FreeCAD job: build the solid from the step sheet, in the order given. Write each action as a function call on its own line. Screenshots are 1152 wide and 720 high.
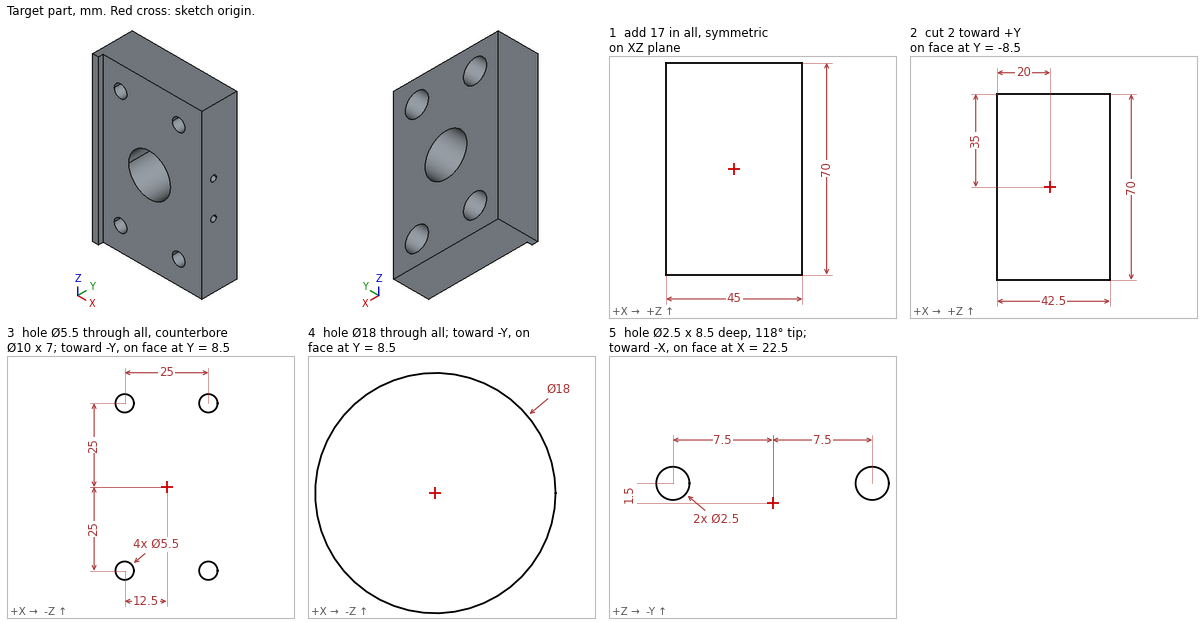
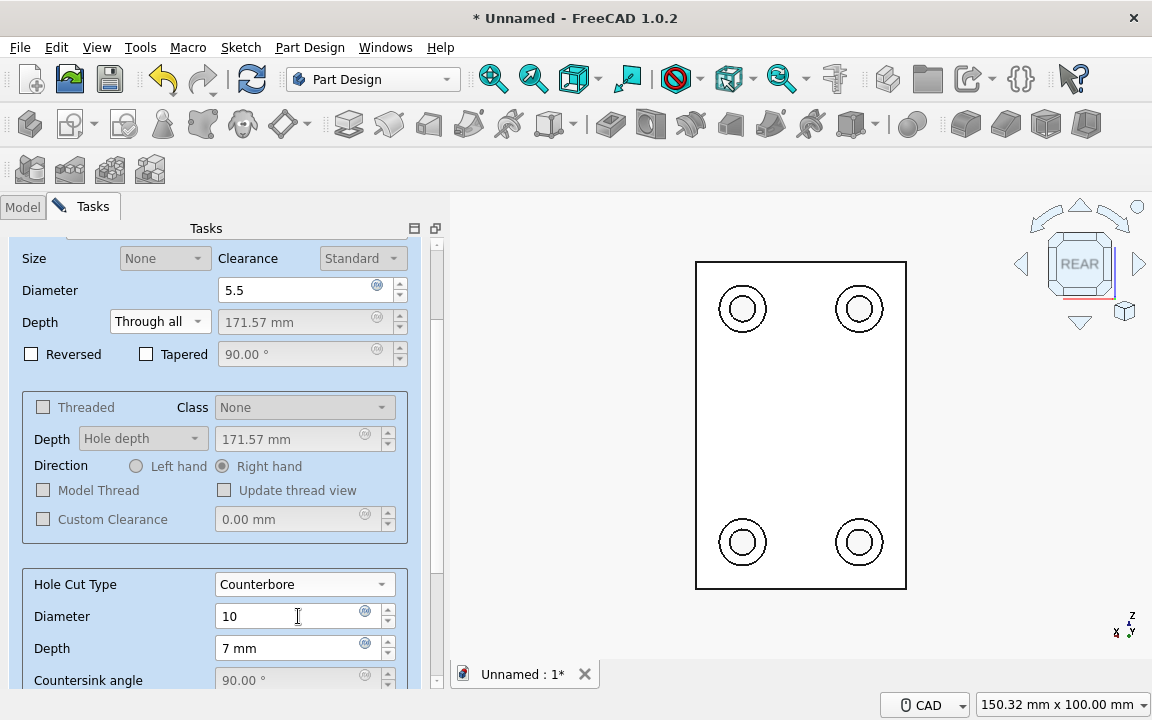
scroll(437, 463, up, 3)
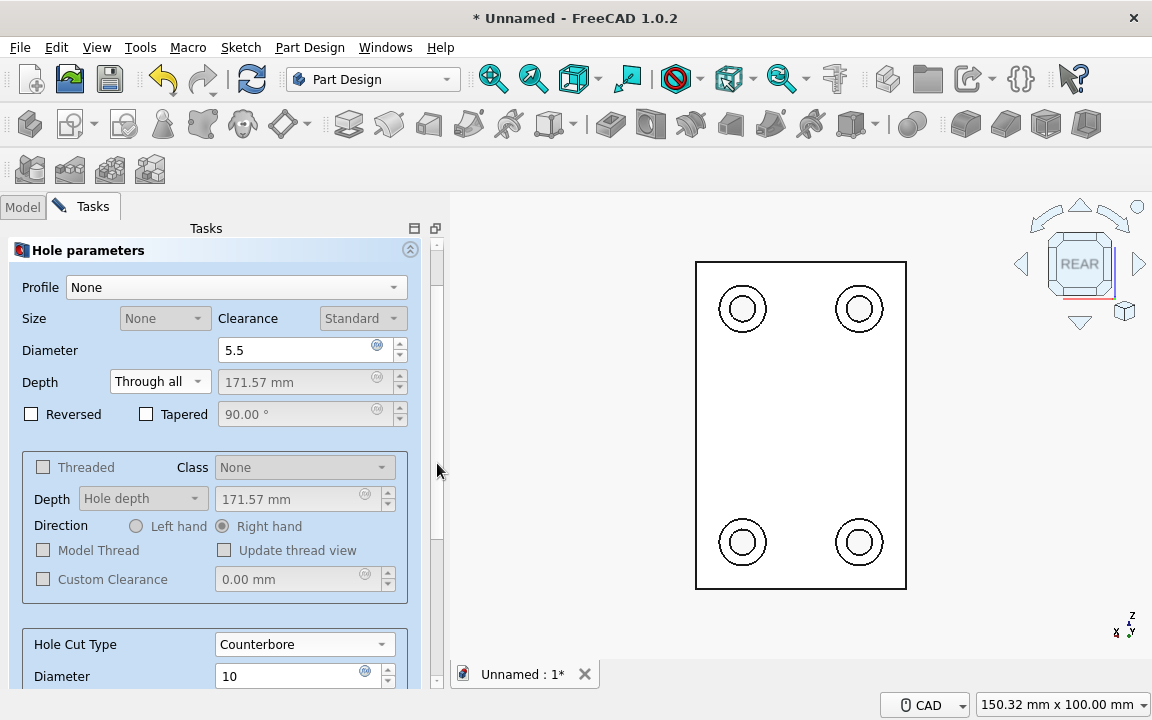
click(167, 267)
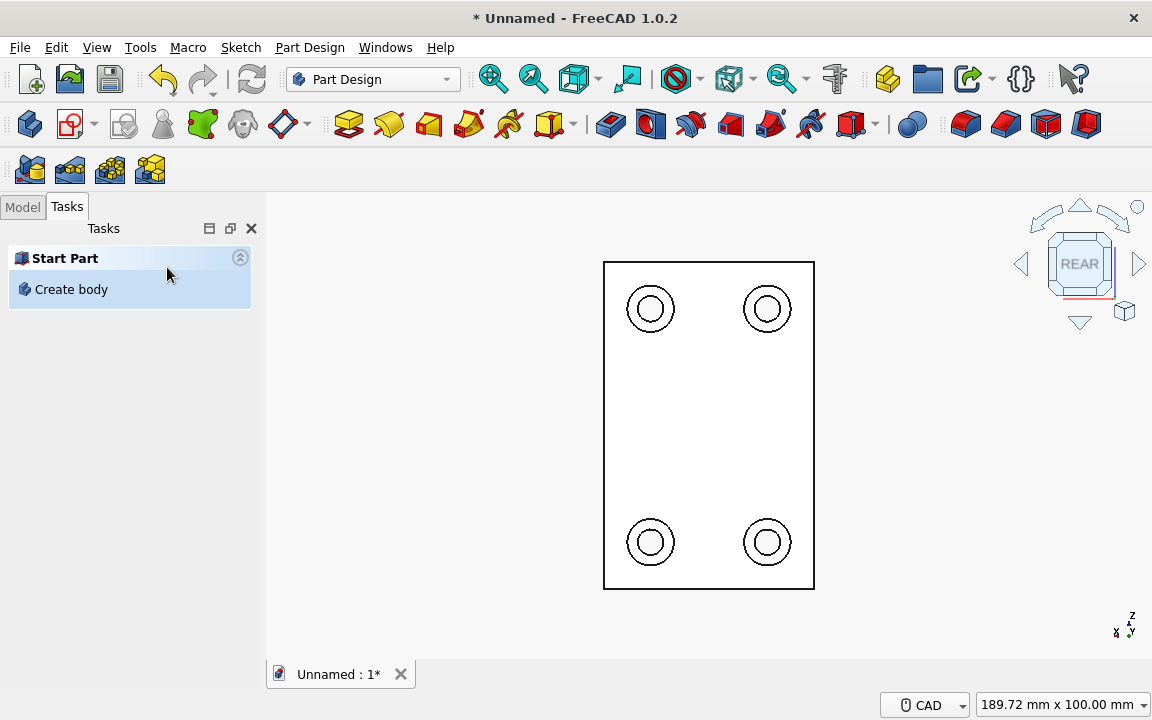
click(709, 424)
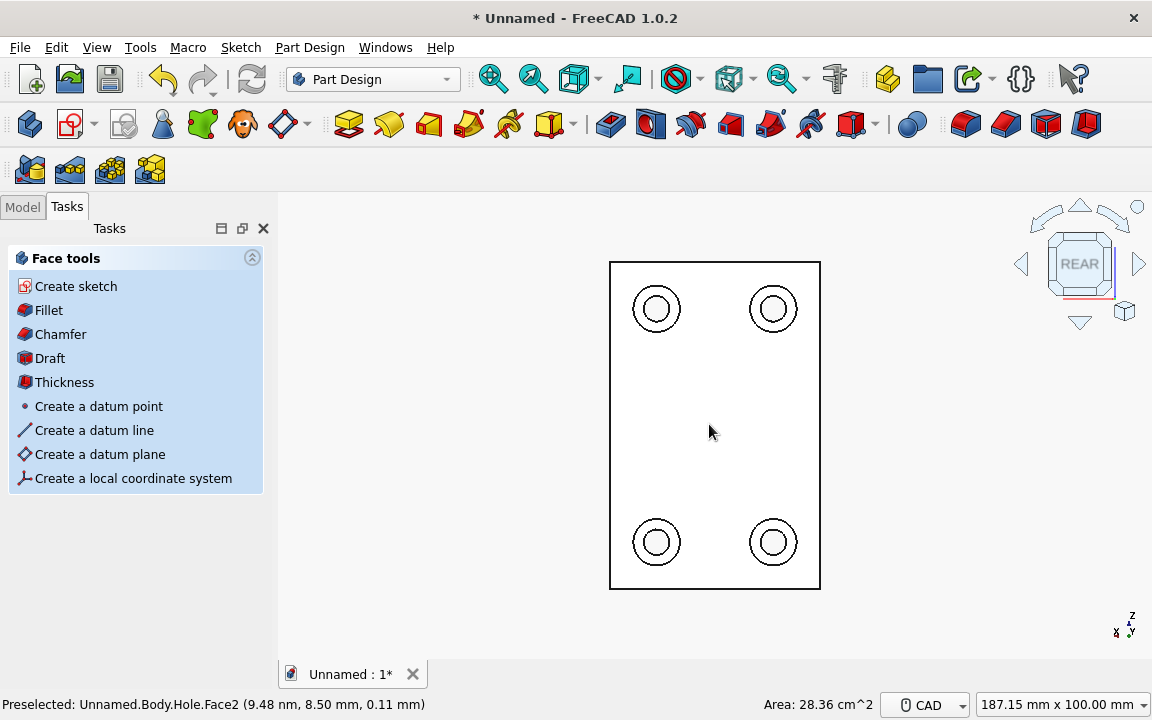
click(70, 124)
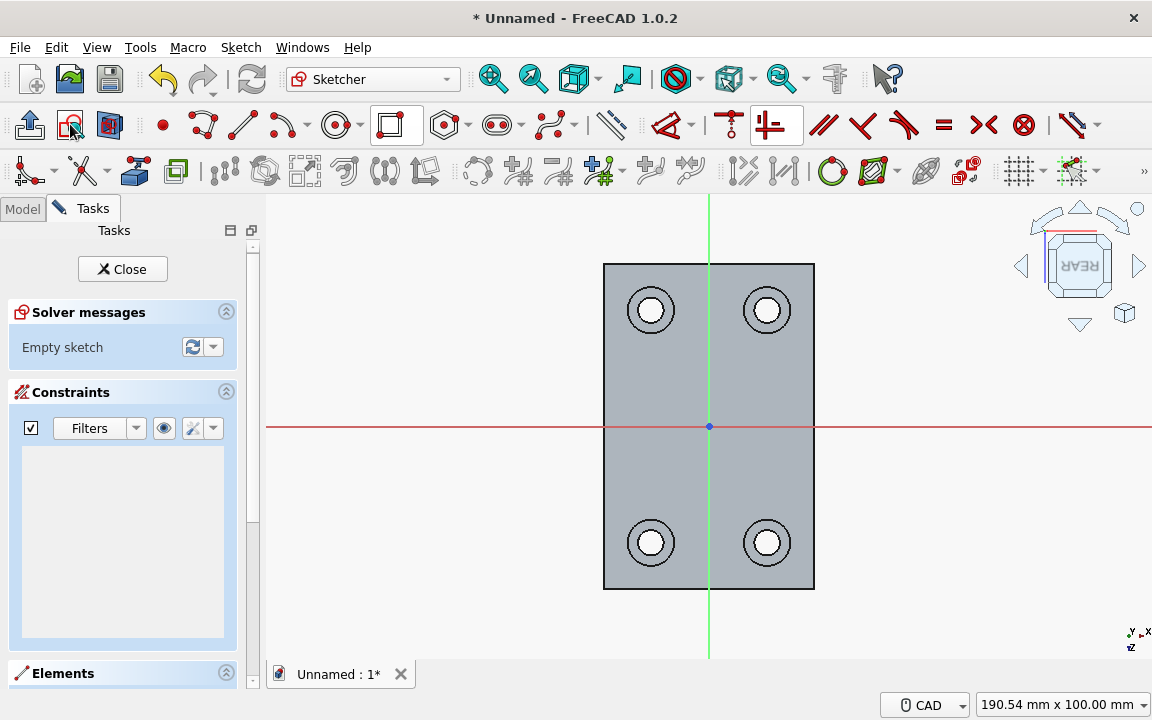
scroll(739, 426, up, 6)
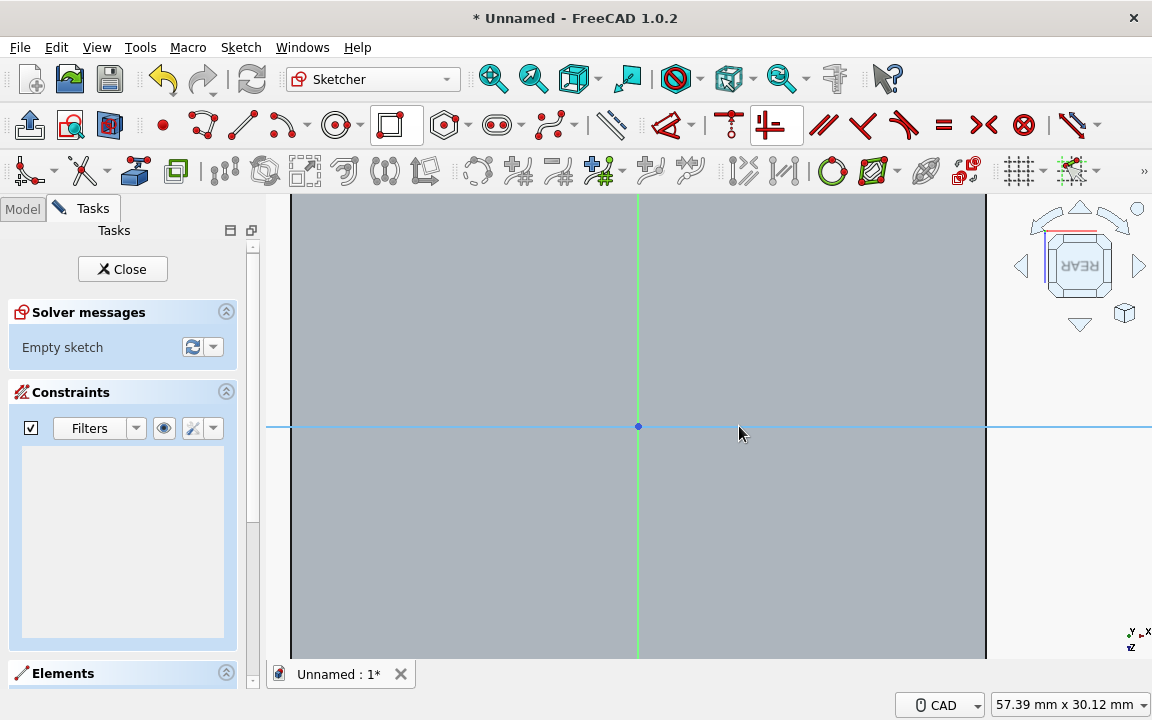
click(336, 126)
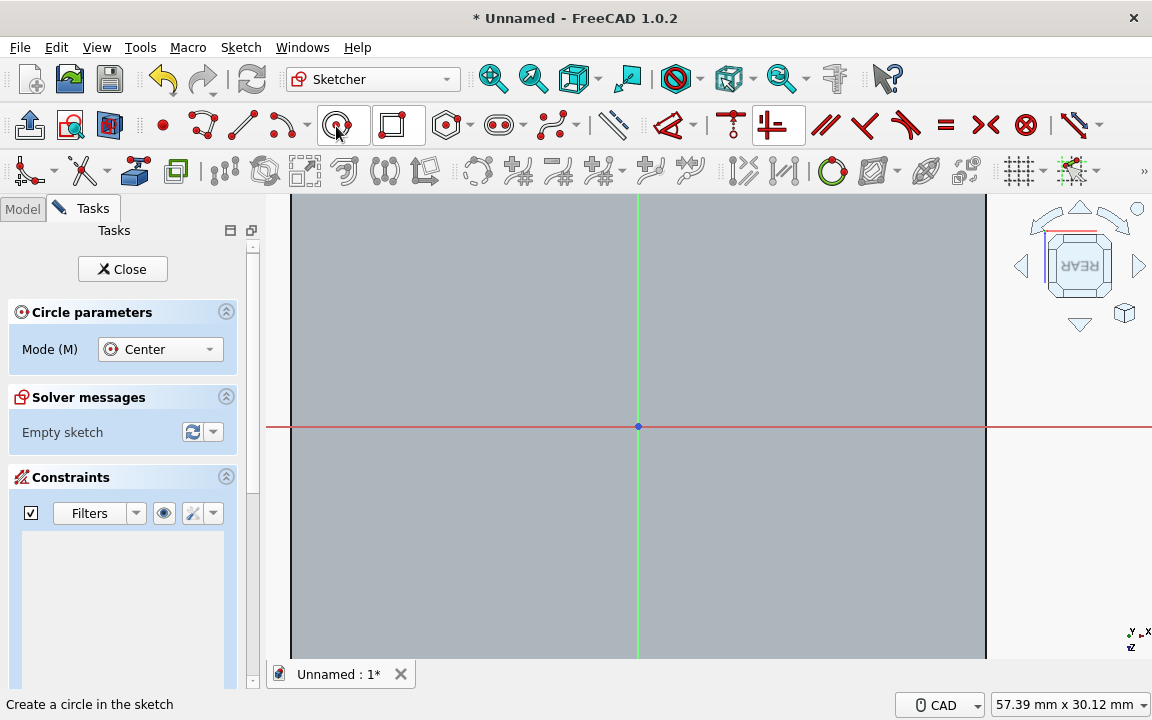
click(638, 426)
move(736, 328)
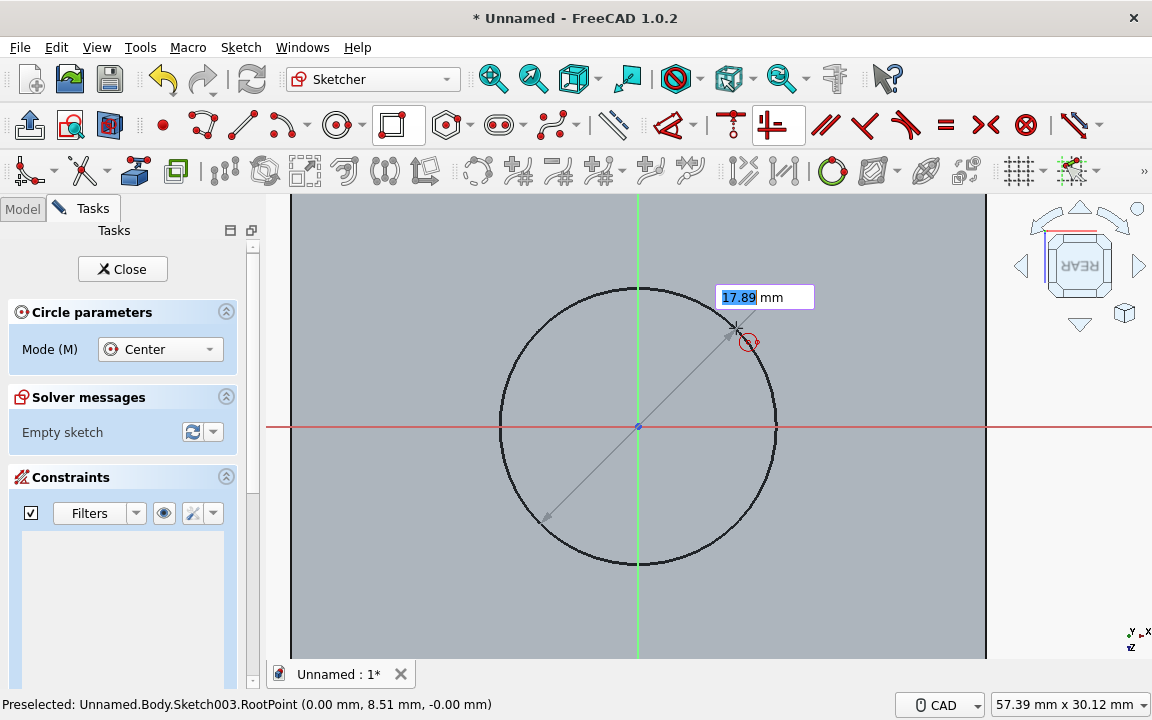
text(18)
key(Return)
key(Escape)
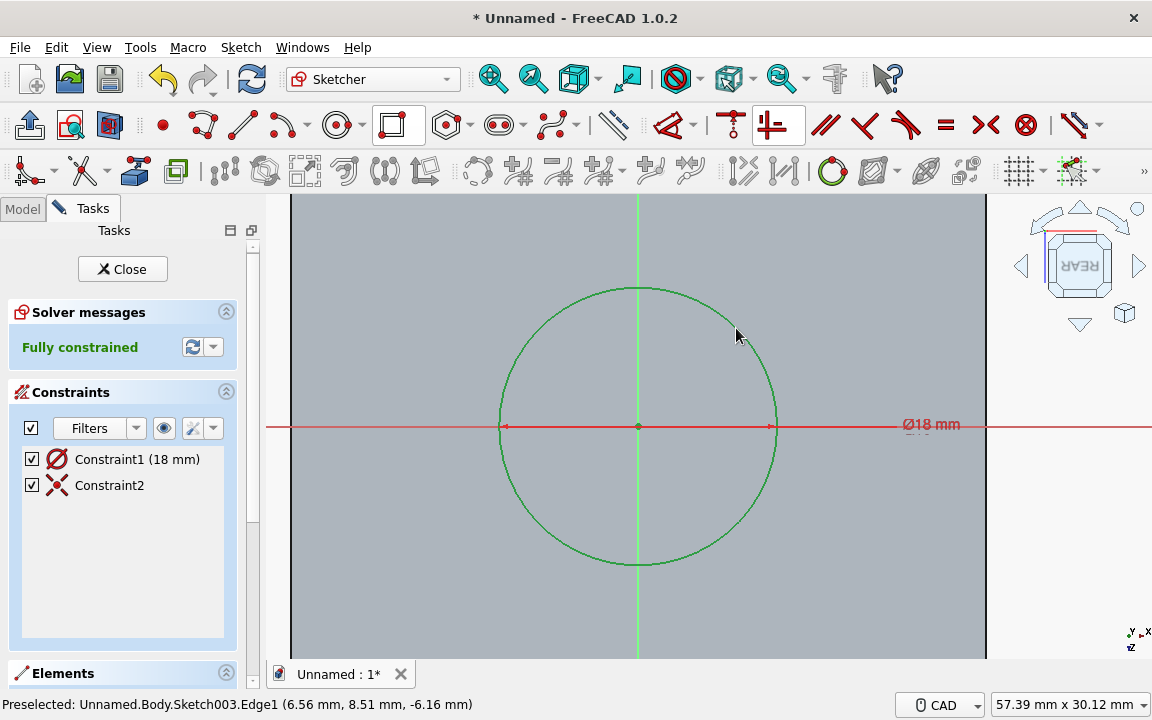
click(123, 269)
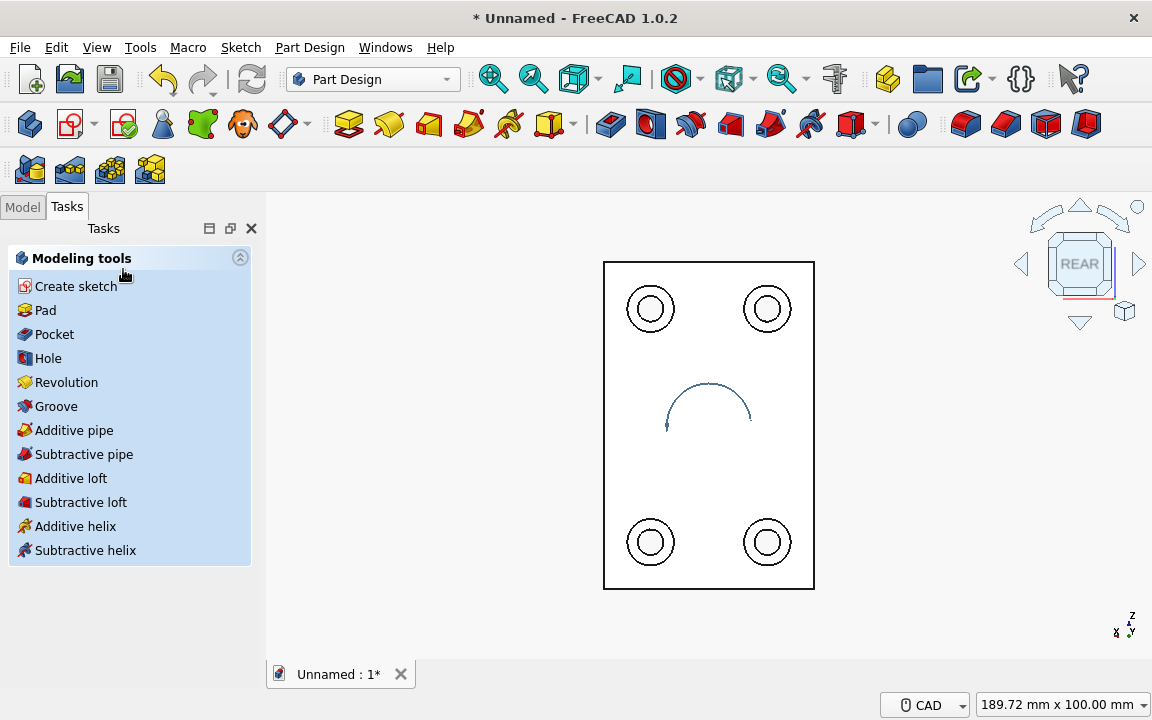
click(652, 124)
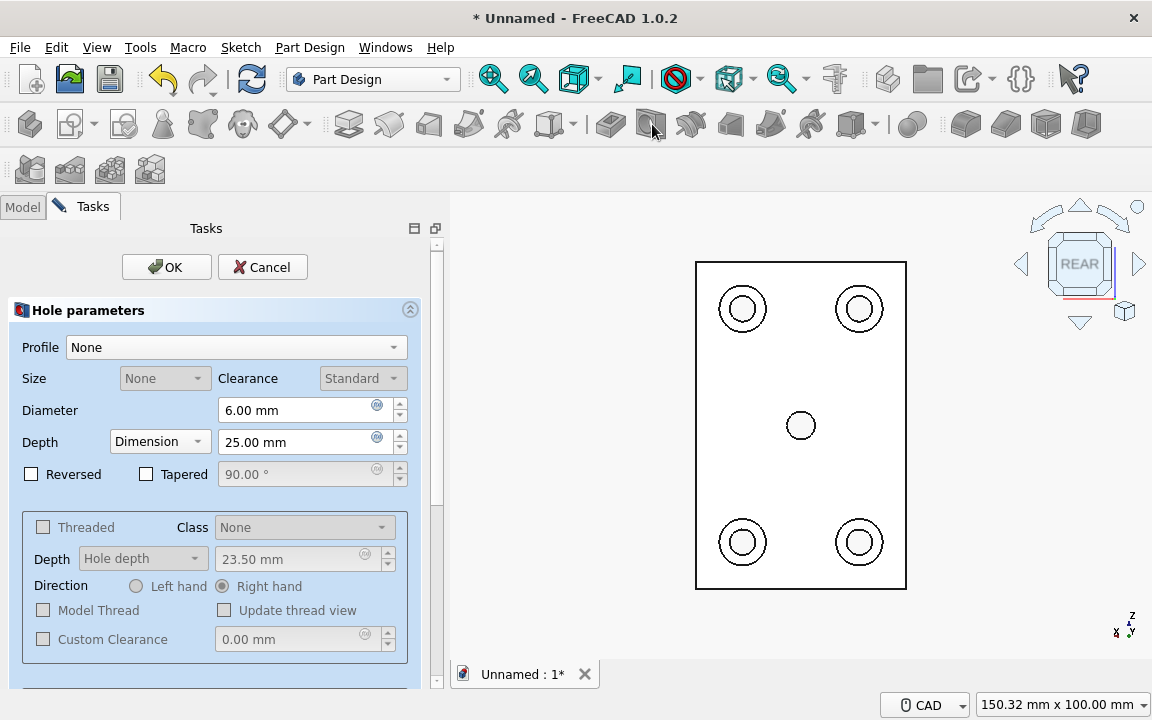
triple_click(305, 410)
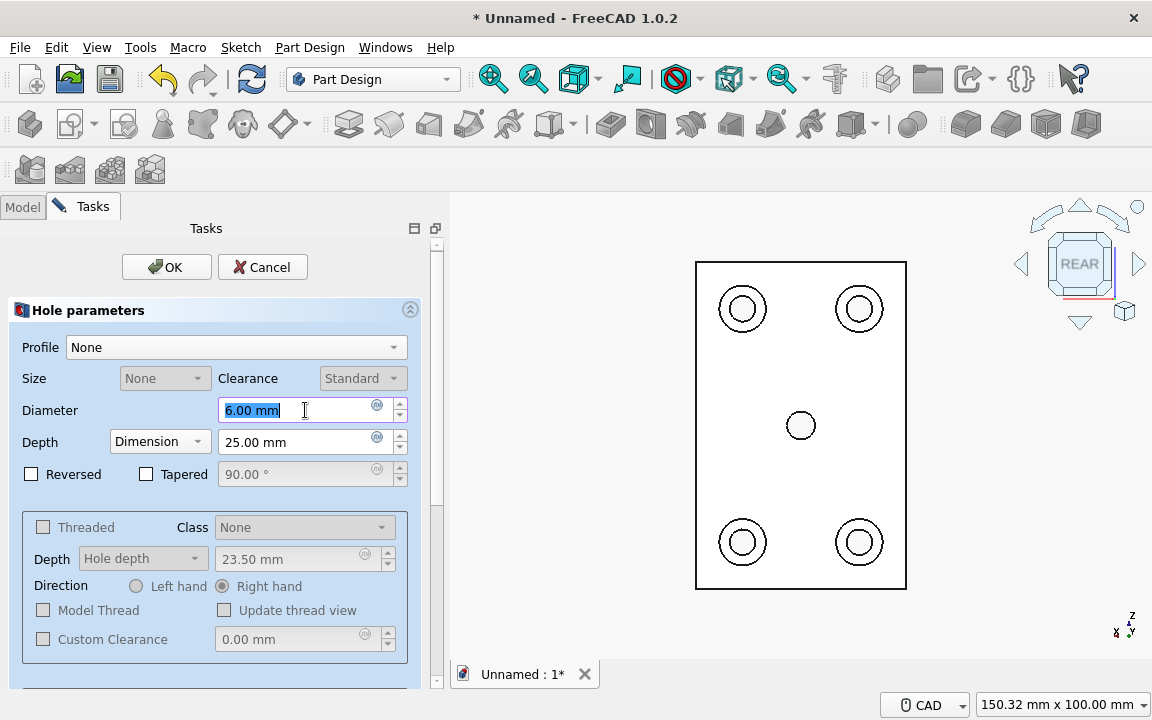
text(18)
key(Tab)